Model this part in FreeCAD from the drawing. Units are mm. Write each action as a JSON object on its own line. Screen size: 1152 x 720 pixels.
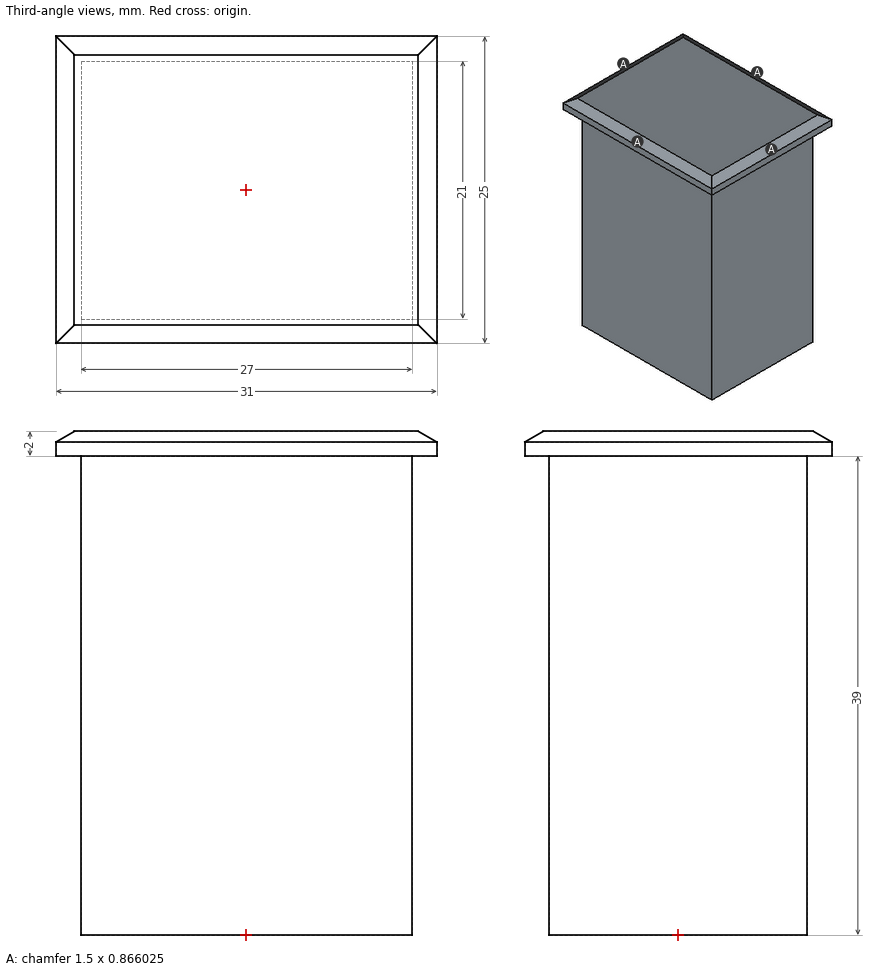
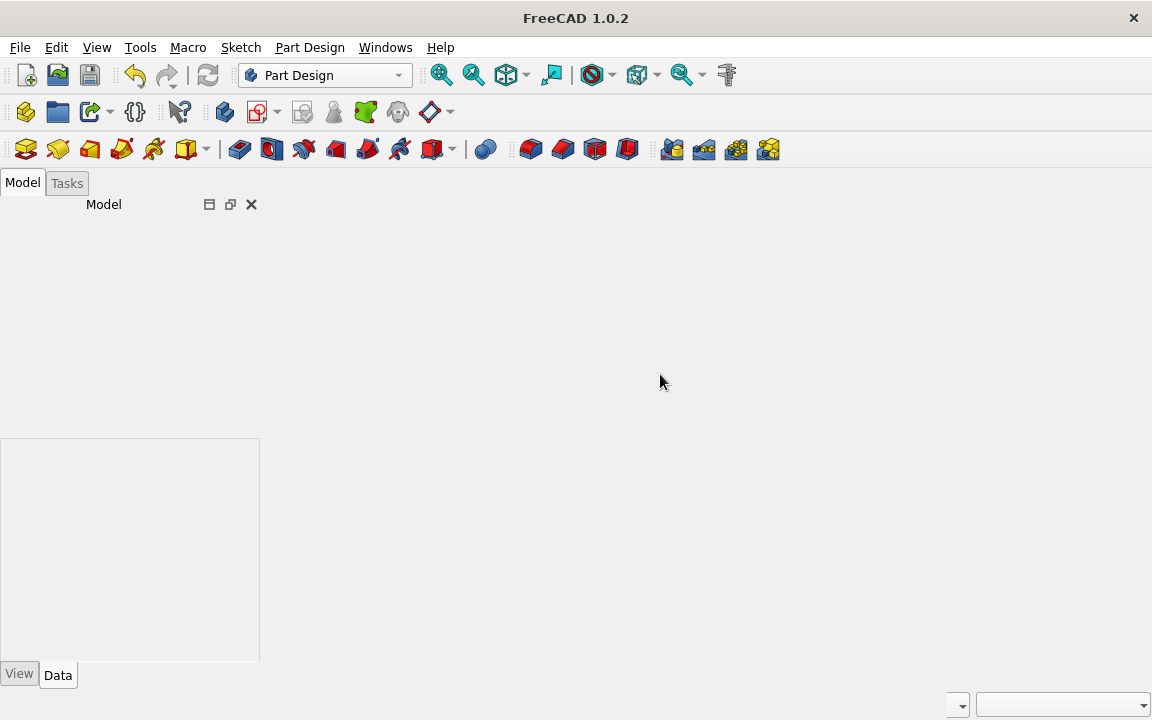
{"action": "key", "text": "ctrl+n"}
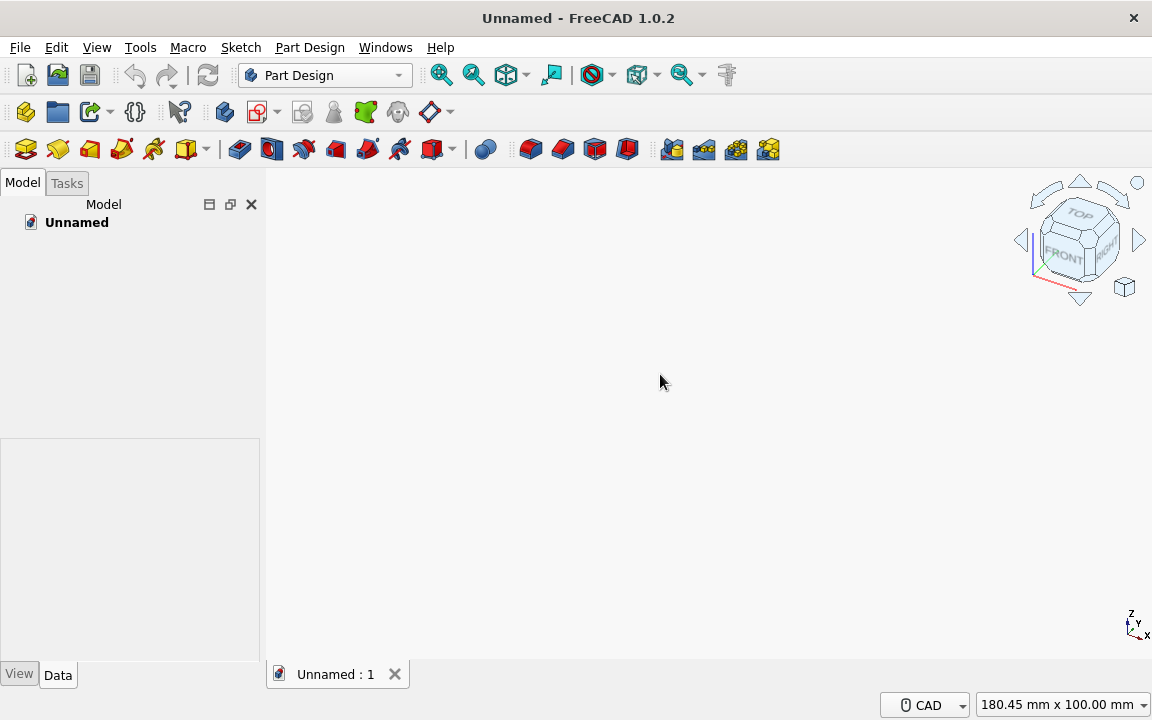
{"action": "left_click", "coordinate": [258, 112]}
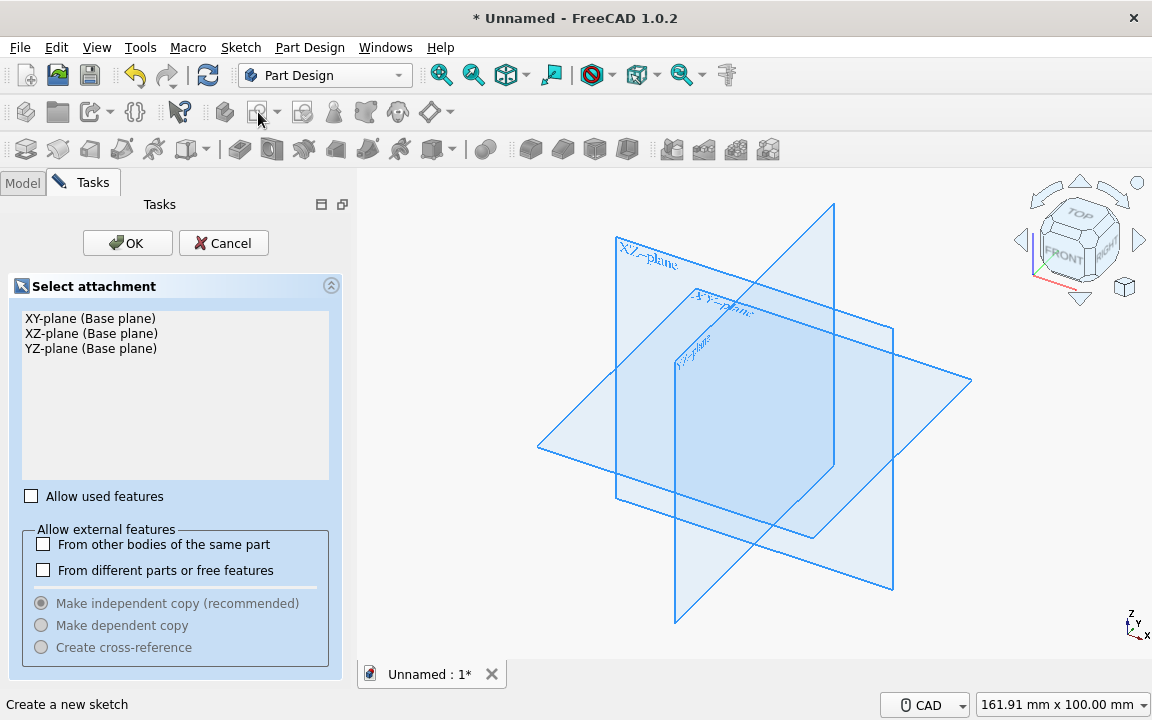
{"action": "left_click", "coordinate": [82, 318]}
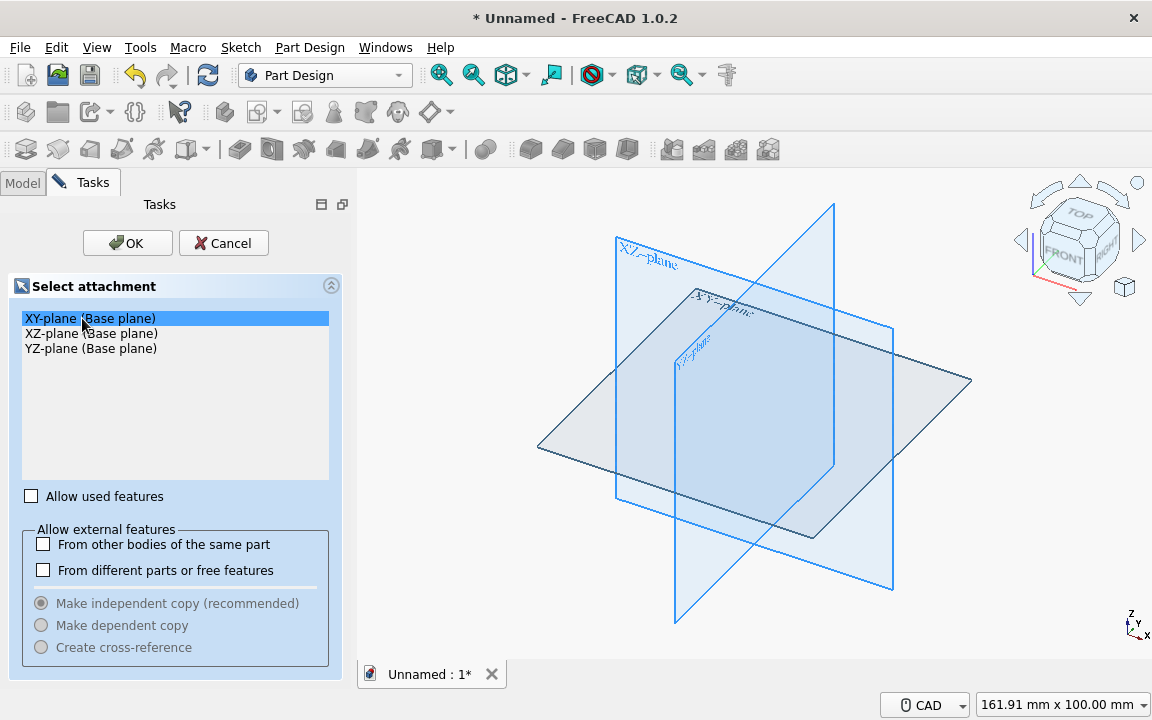
{"action": "left_click", "coordinate": [128, 243]}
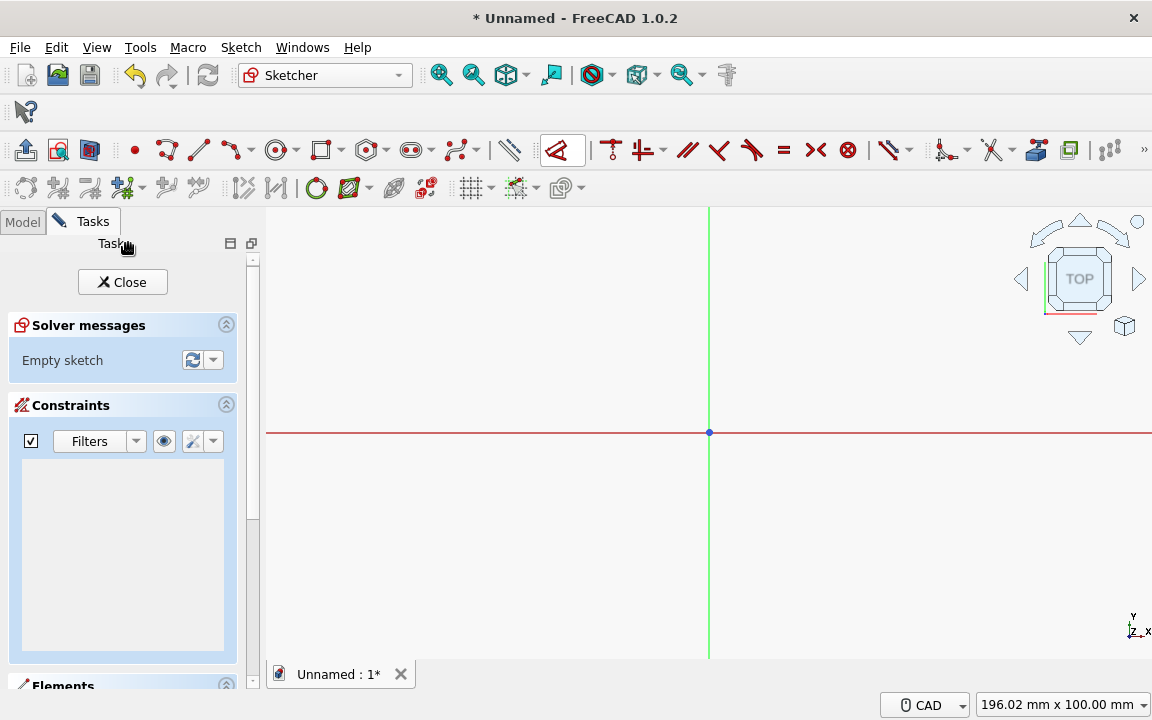
{"action": "scroll", "coordinate": [749, 433], "scroll_direction": "up", "scroll_amount": 5}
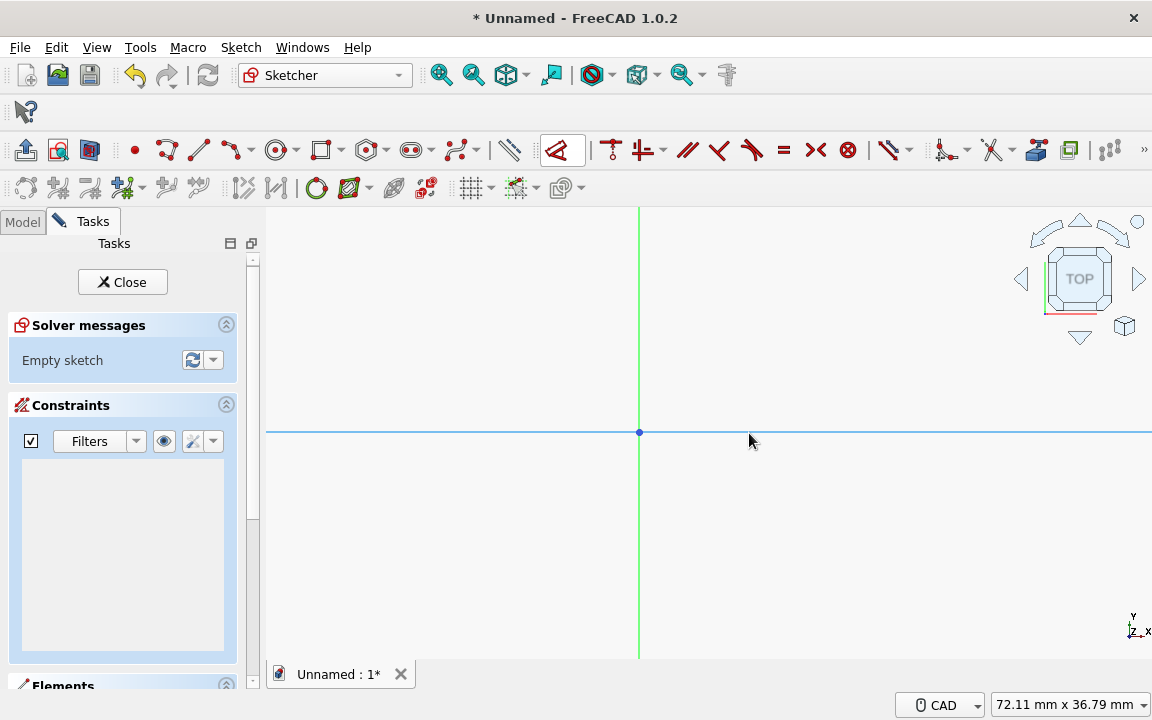
{"action": "left_click", "coordinate": [344, 150]}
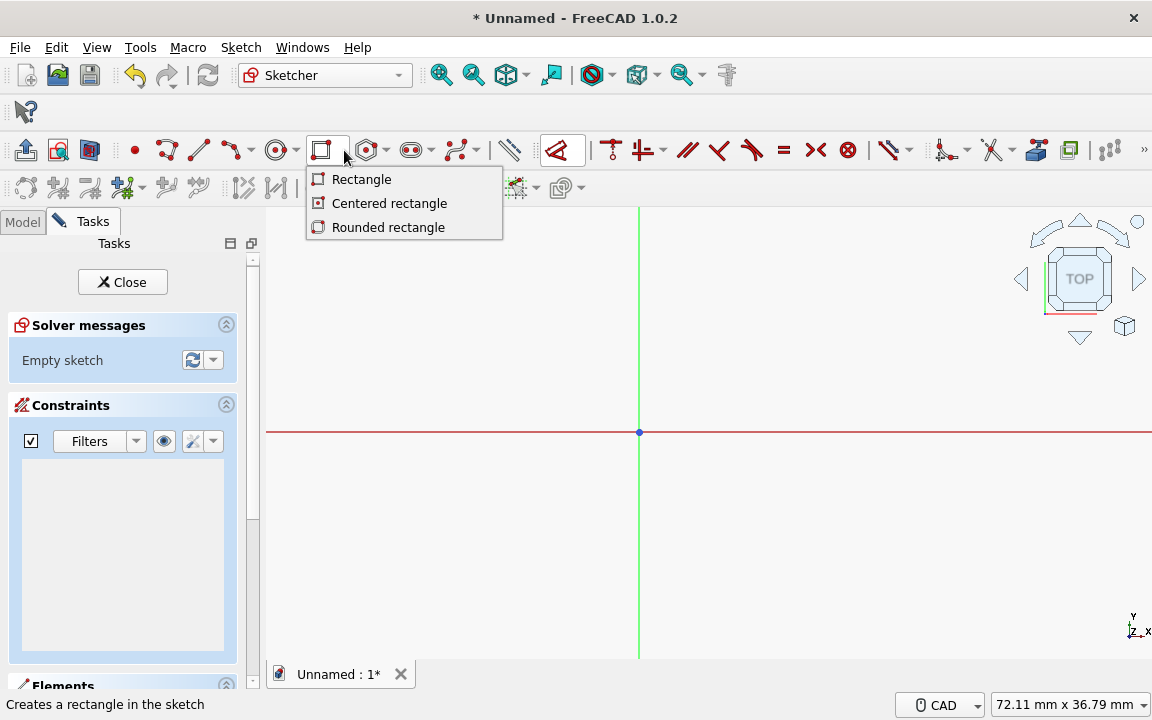
{"action": "left_click", "coordinate": [404, 203]}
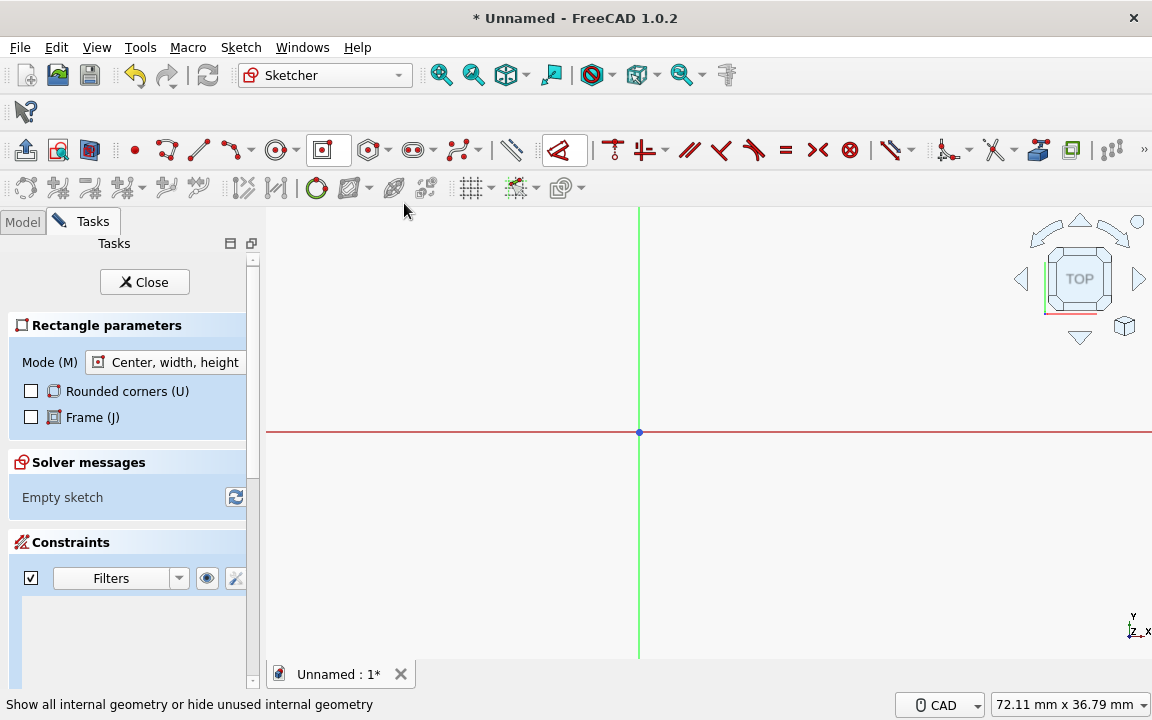
{"action": "left_click", "coordinate": [639, 432]}
{"action": "mouse_move", "coordinate": [805, 303]}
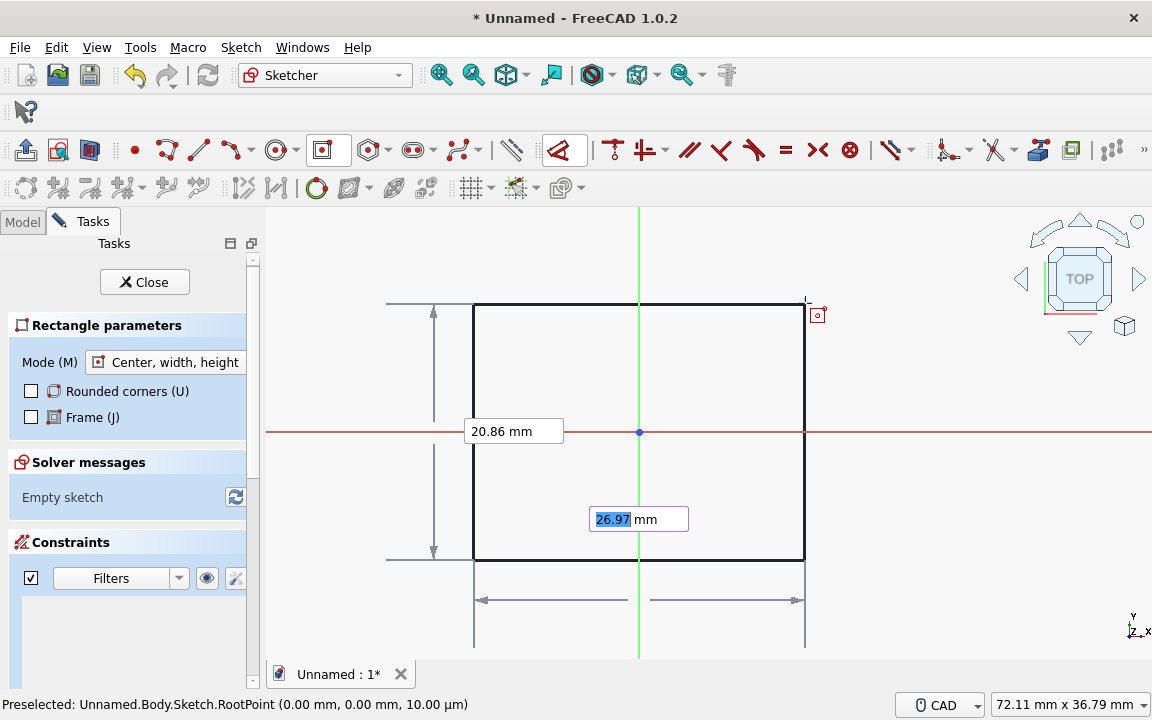
{"action": "type", "text": "27"}
{"action": "key", "text": "Tab"}
{"action": "type", "text": "21"}
{"action": "key", "text": "Return"}
{"action": "key", "text": "Escape"}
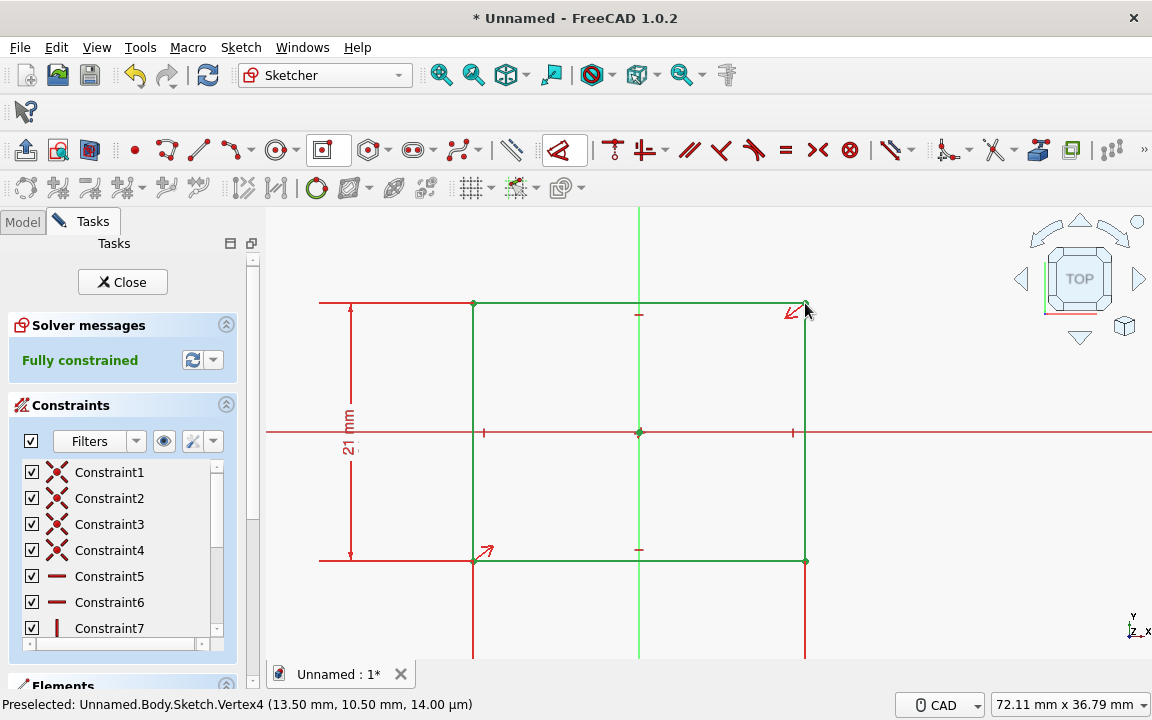
{"action": "left_click", "coordinate": [123, 282]}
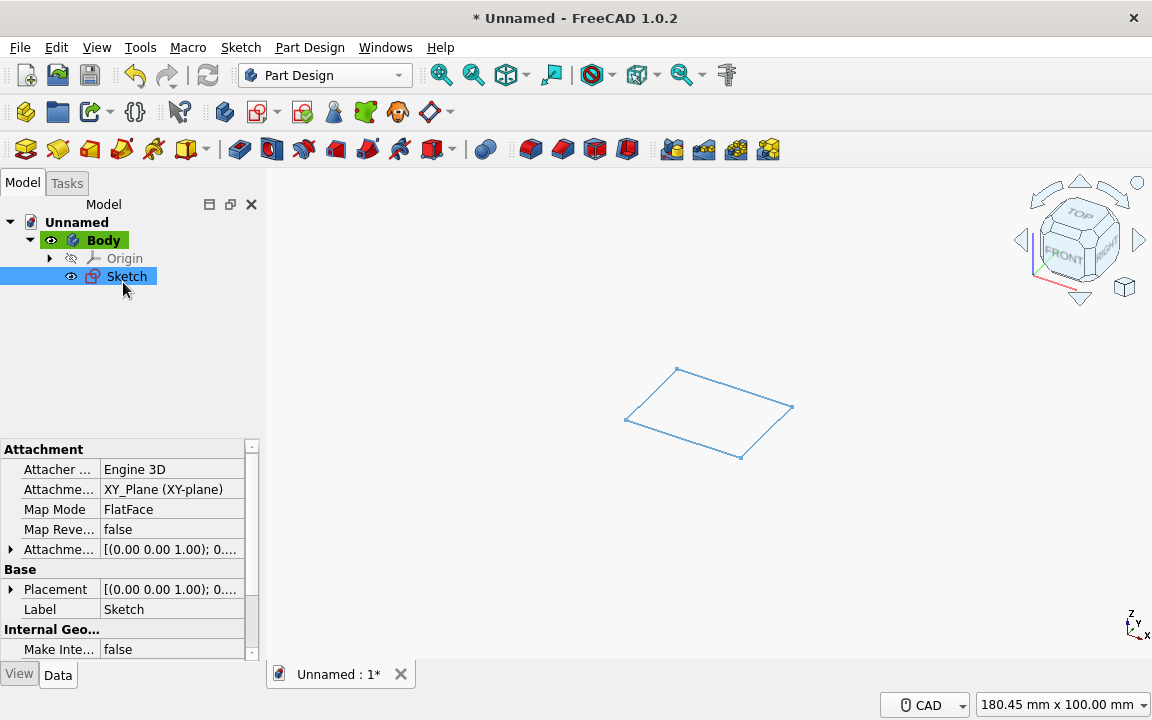
{"action": "left_click", "coordinate": [26, 150]}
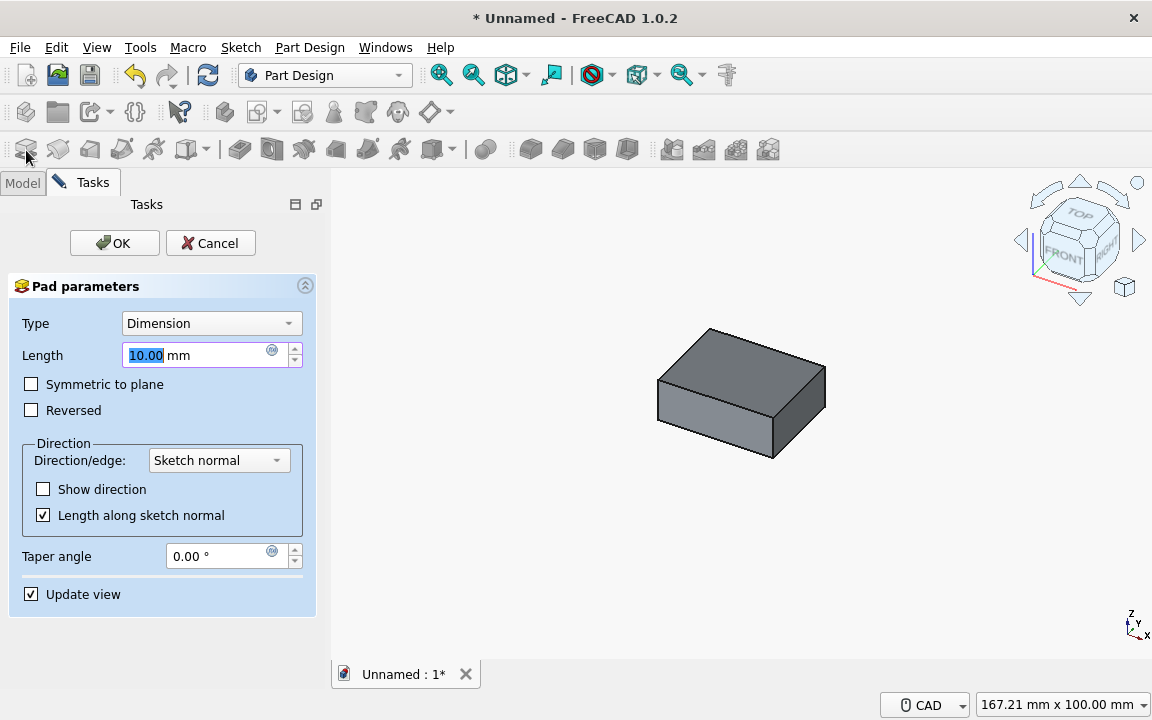
{"action": "type", "text": "39"}
{"action": "key", "text": "Tab"}